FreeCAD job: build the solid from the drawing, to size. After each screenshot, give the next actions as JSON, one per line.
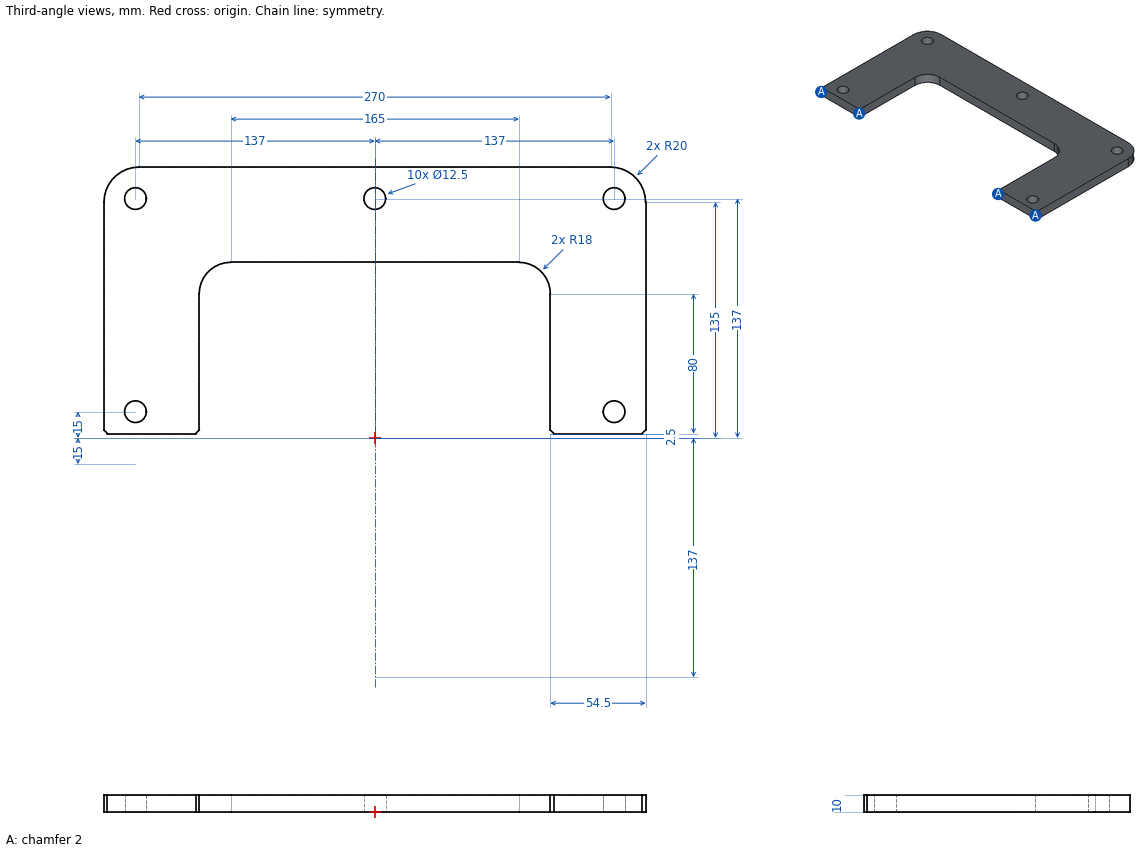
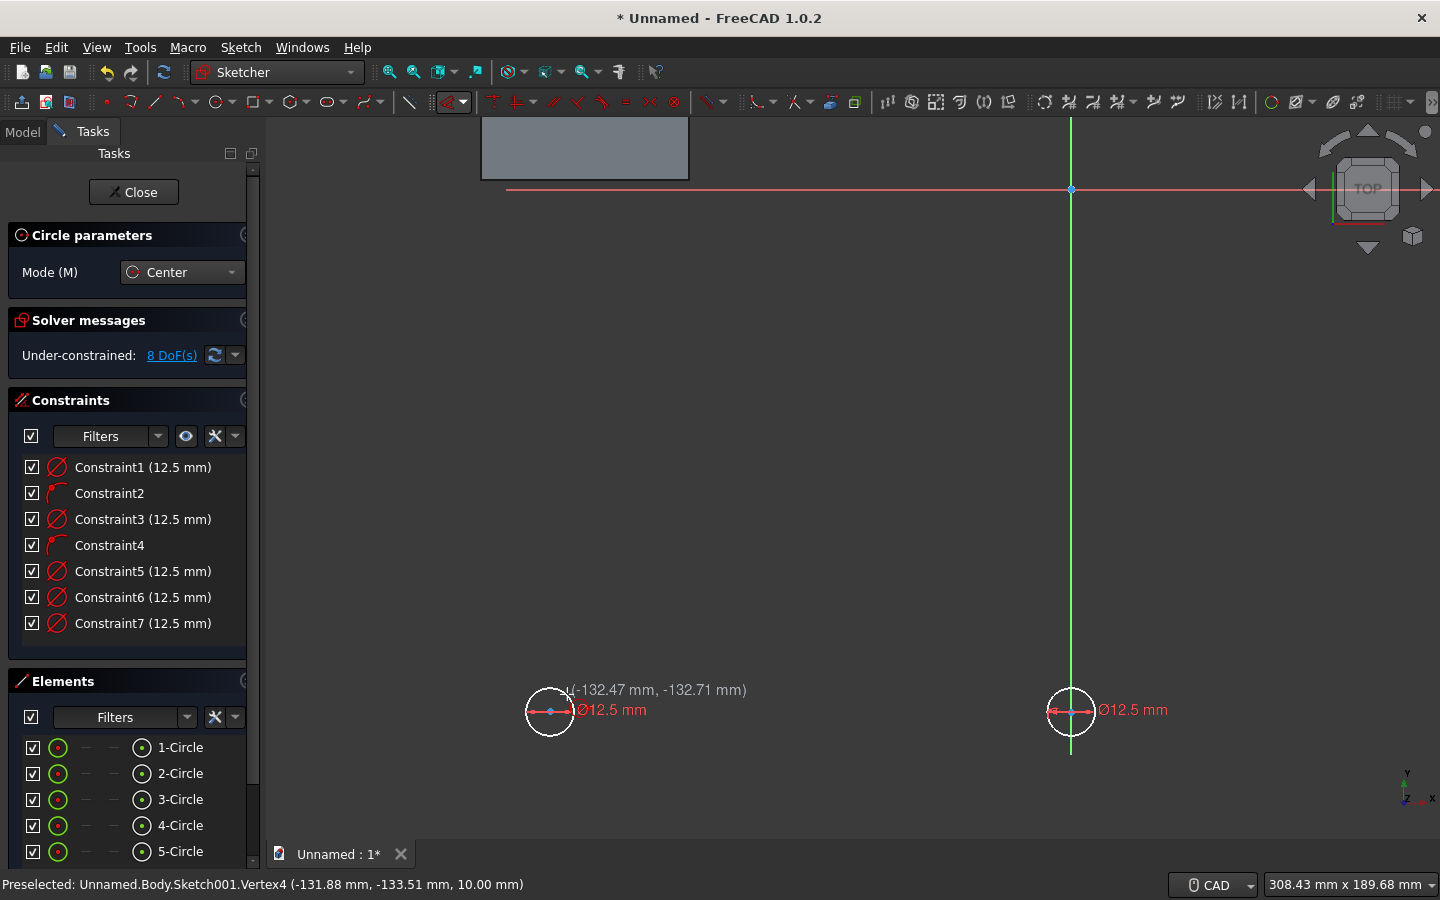
{"action": "scroll", "coordinate": [551, 713], "scroll_direction": "down", "scroll_amount": 4}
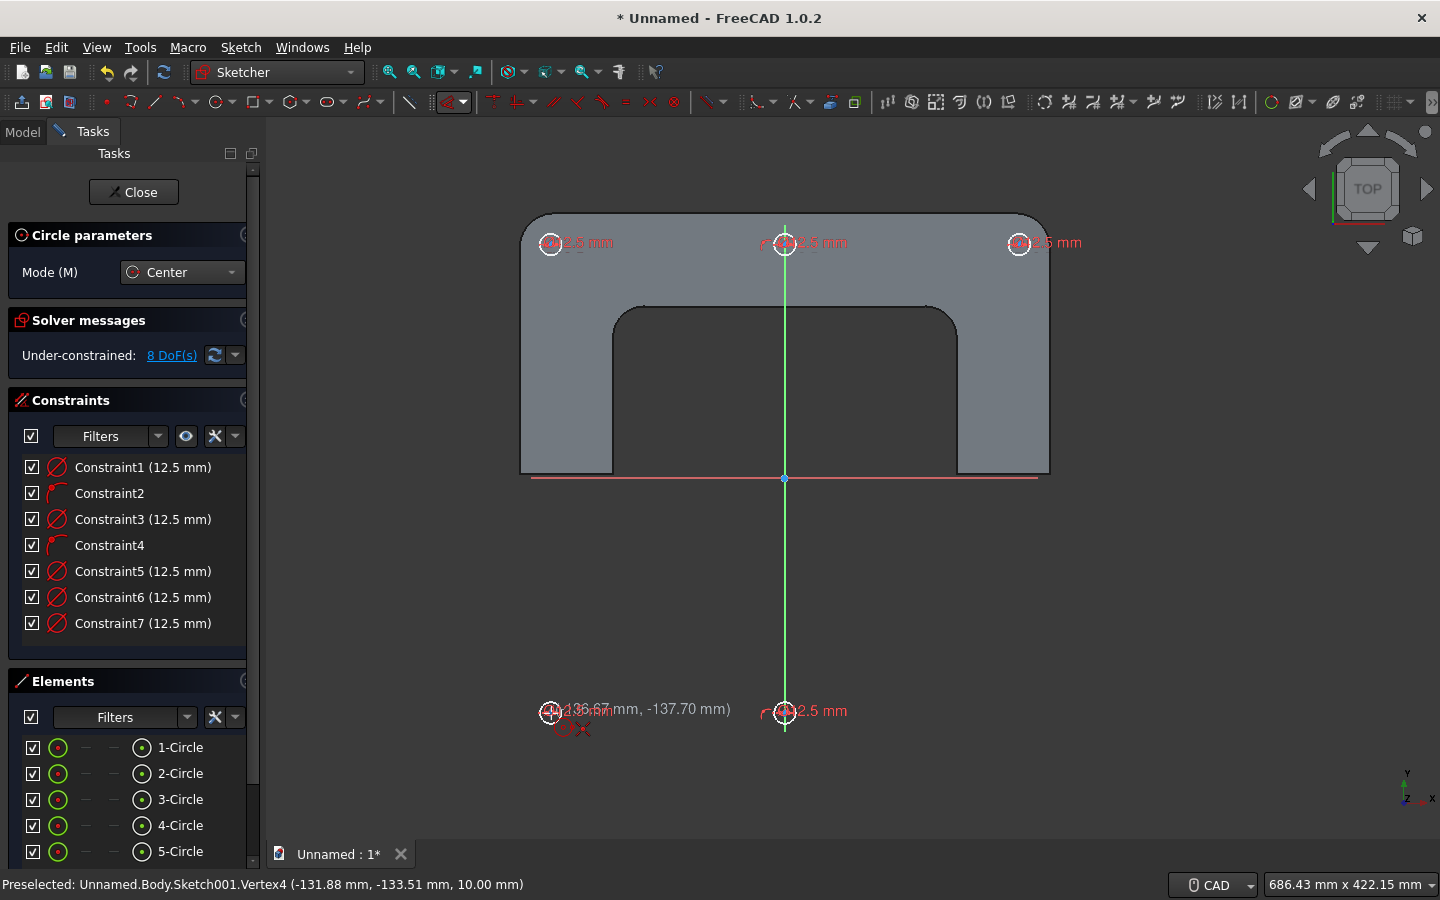
{"action": "scroll", "coordinate": [1019, 713], "scroll_direction": "up", "scroll_amount": 4}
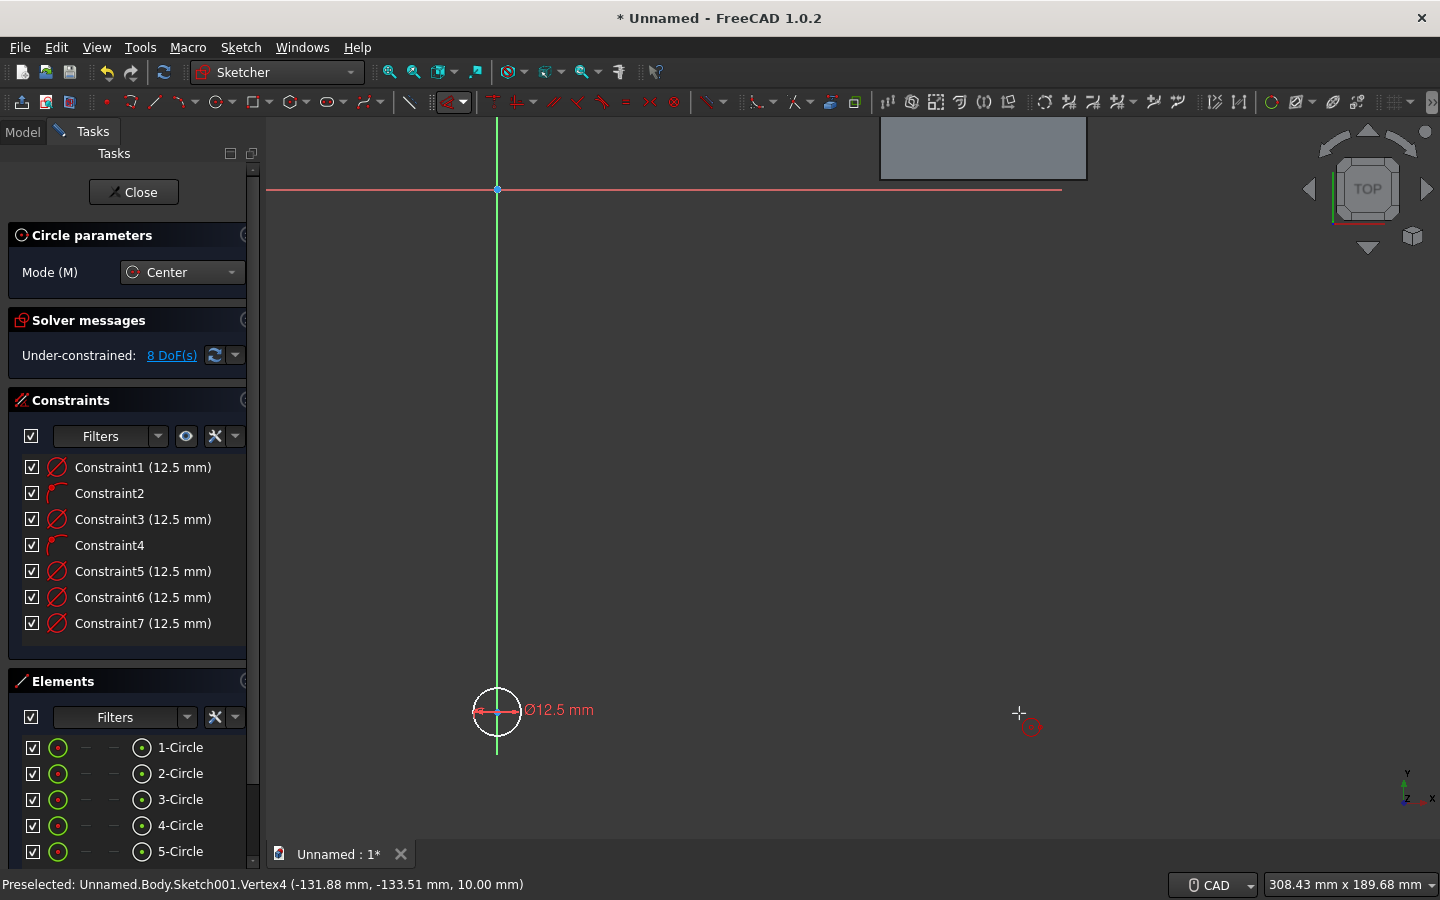
{"action": "left_click", "coordinate": [1019, 711]}
{"action": "mouse_move", "coordinate": [1035, 694]}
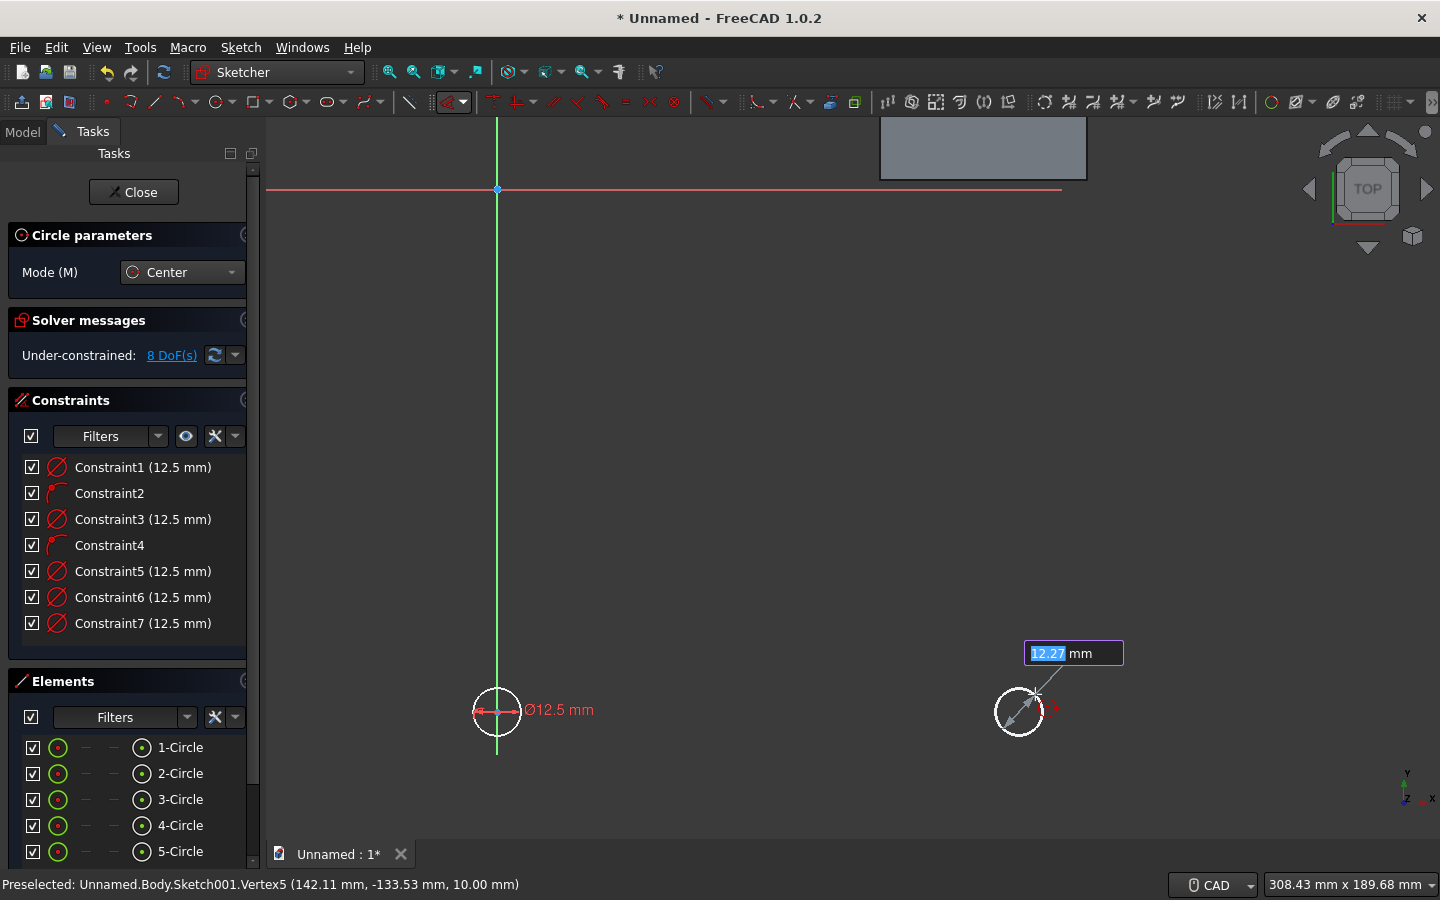
{"action": "type", "text": "12.5"}
{"action": "key", "text": "Return"}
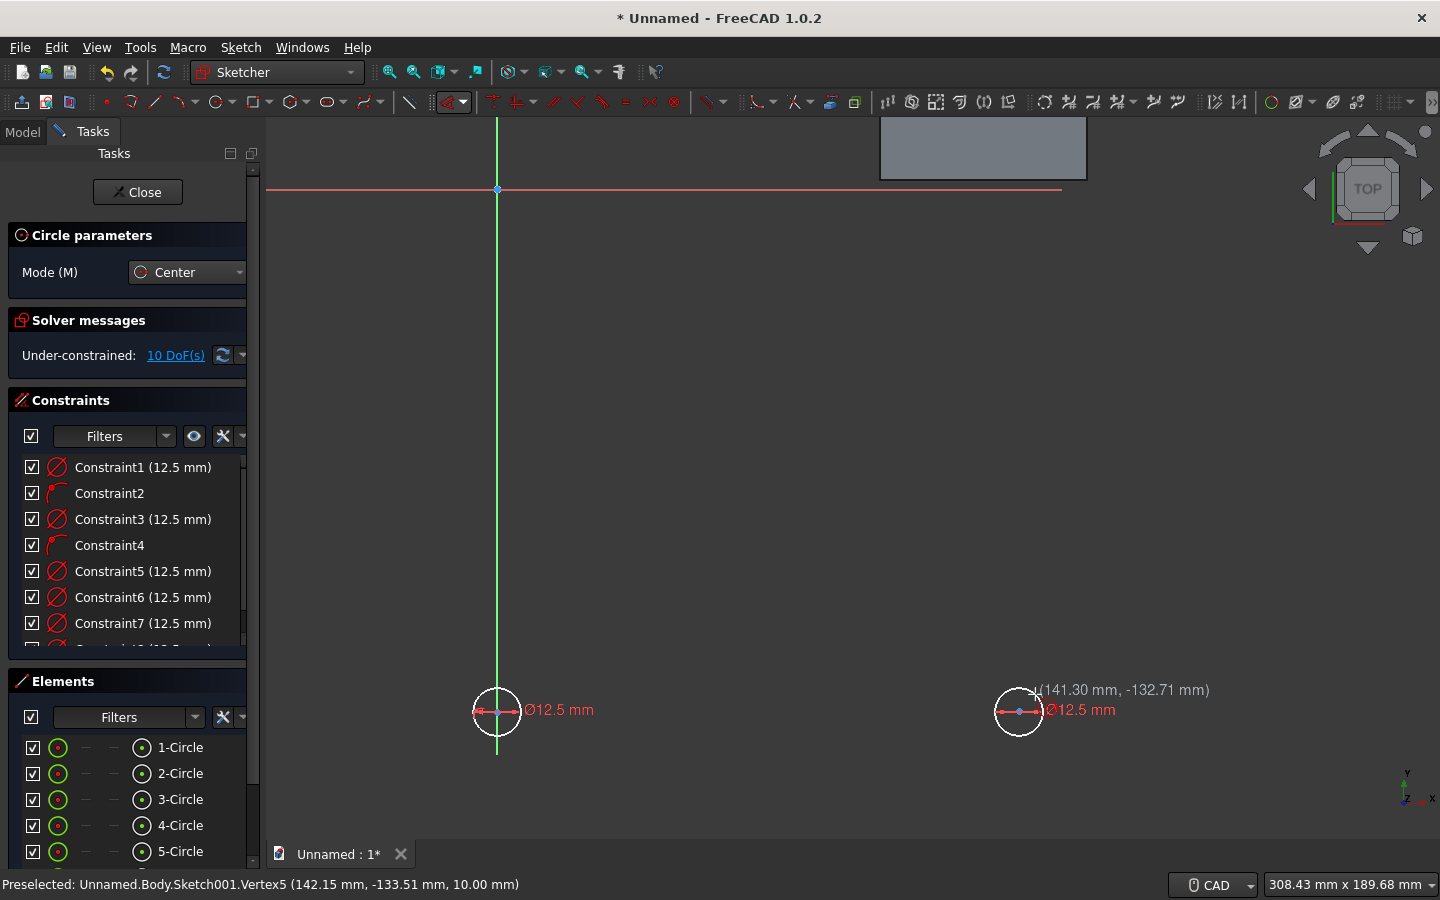
{"action": "scroll", "coordinate": [1019, 713], "scroll_direction": "down", "scroll_amount": 4}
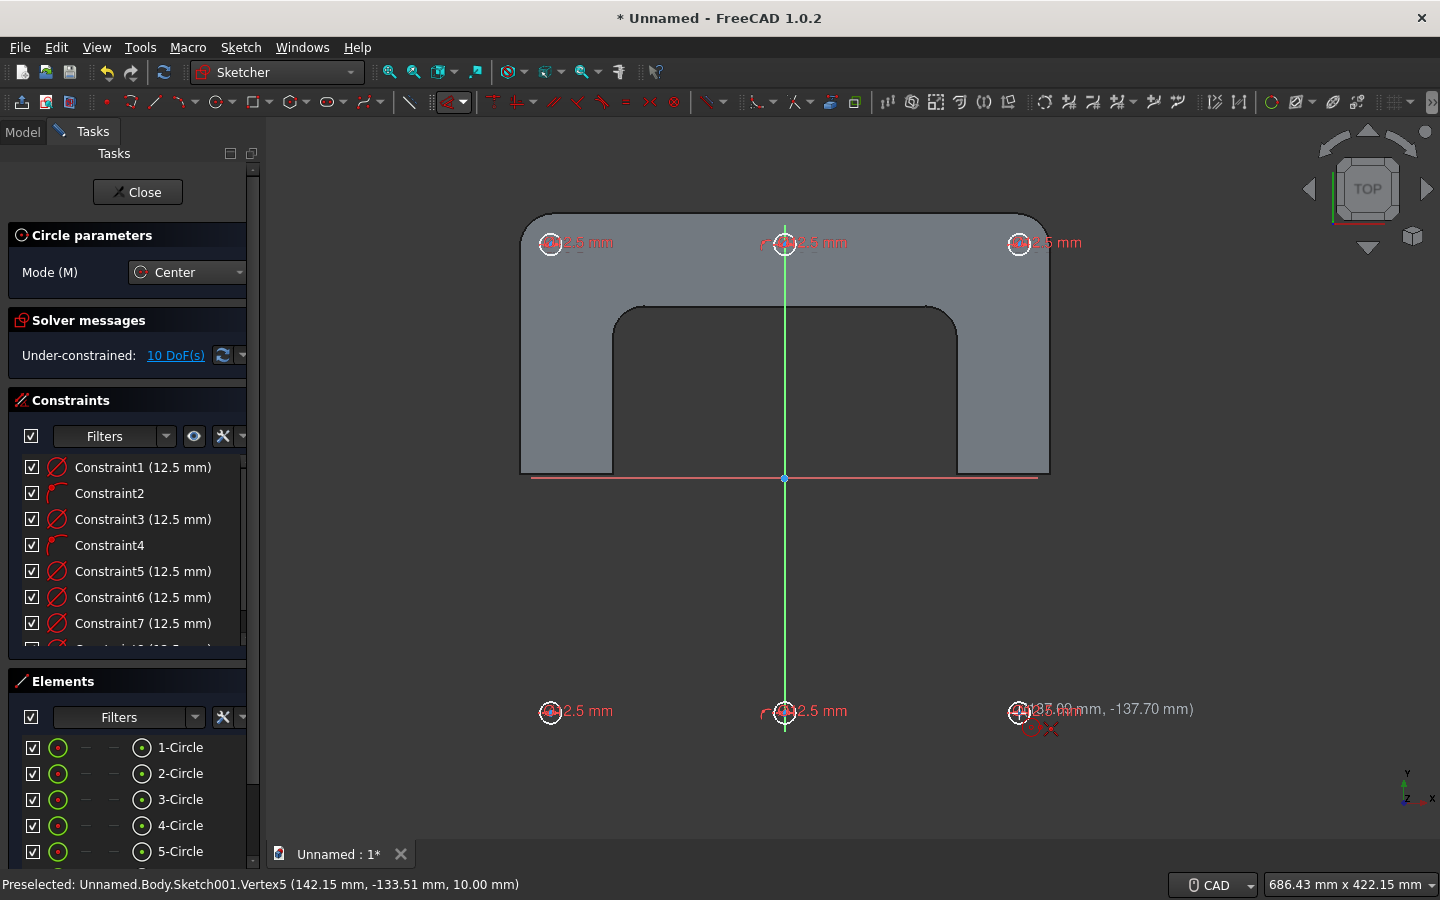
{"action": "scroll", "coordinate": [551, 453], "scroll_direction": "up", "scroll_amount": 4}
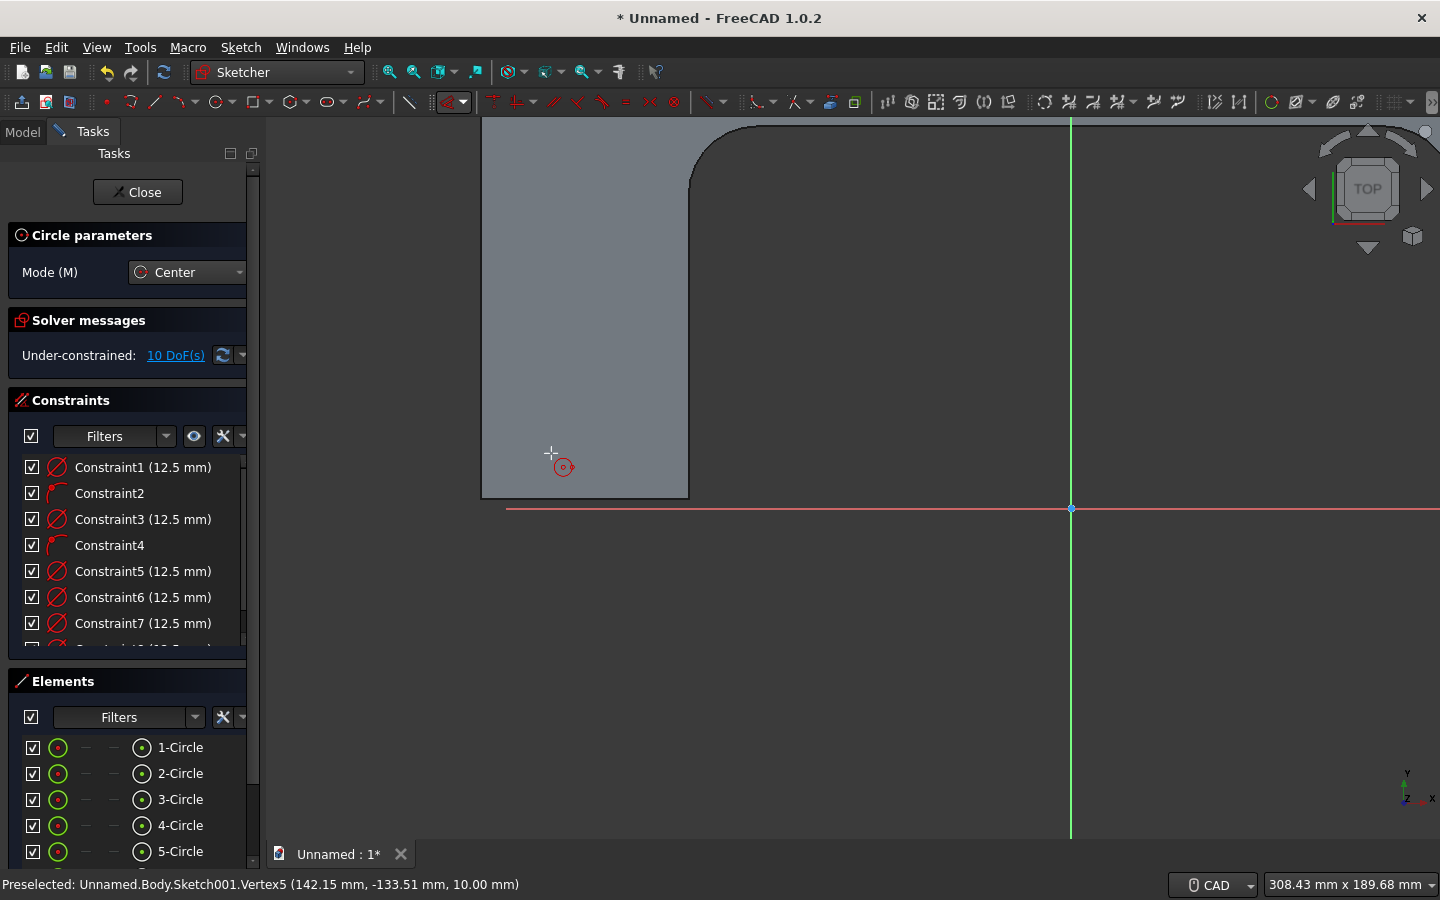
{"action": "left_click", "coordinate": [550, 452]}
{"action": "mouse_move", "coordinate": [567, 435]}